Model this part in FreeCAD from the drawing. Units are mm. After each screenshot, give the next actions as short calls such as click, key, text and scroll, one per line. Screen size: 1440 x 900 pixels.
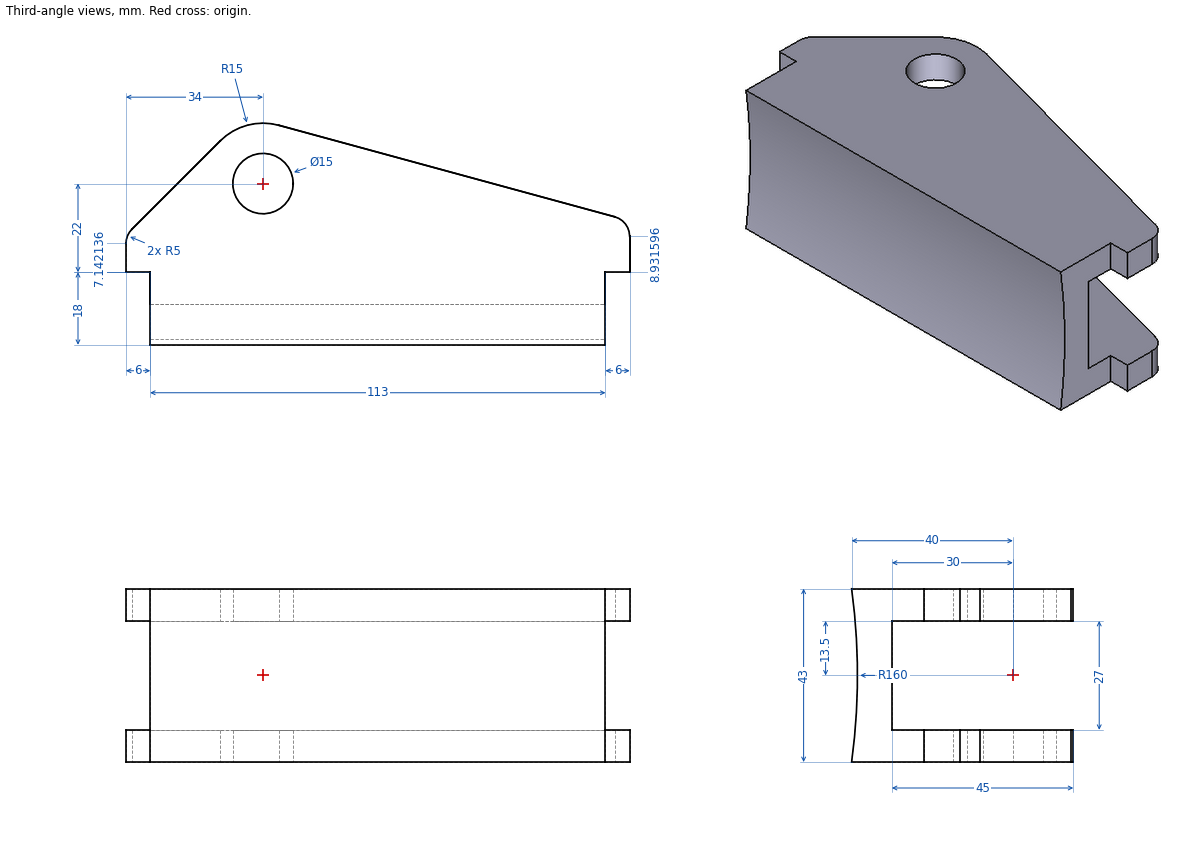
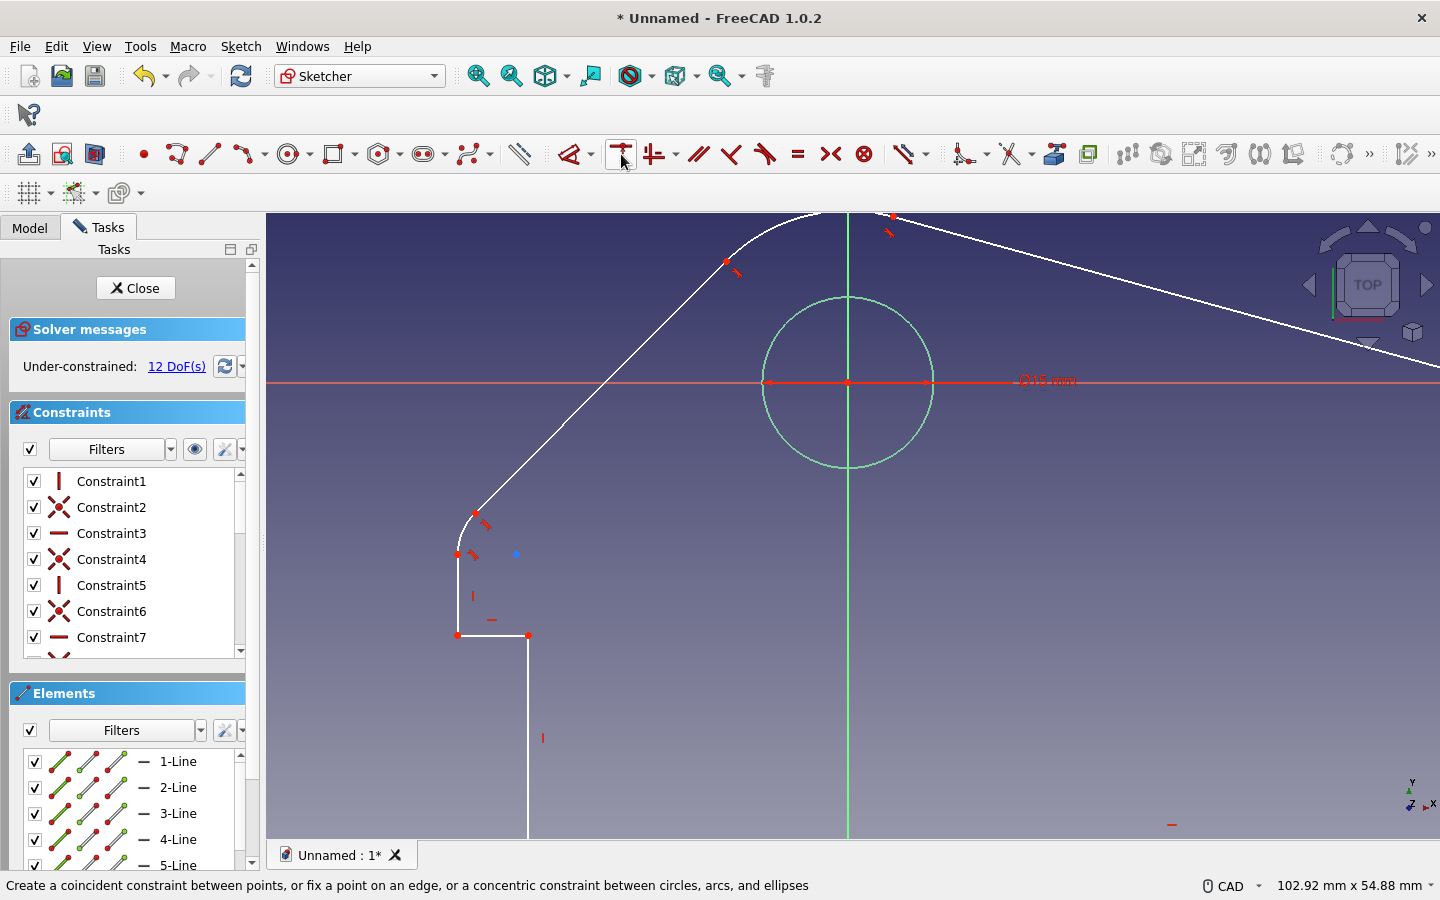
scroll(468, 524, down, 4)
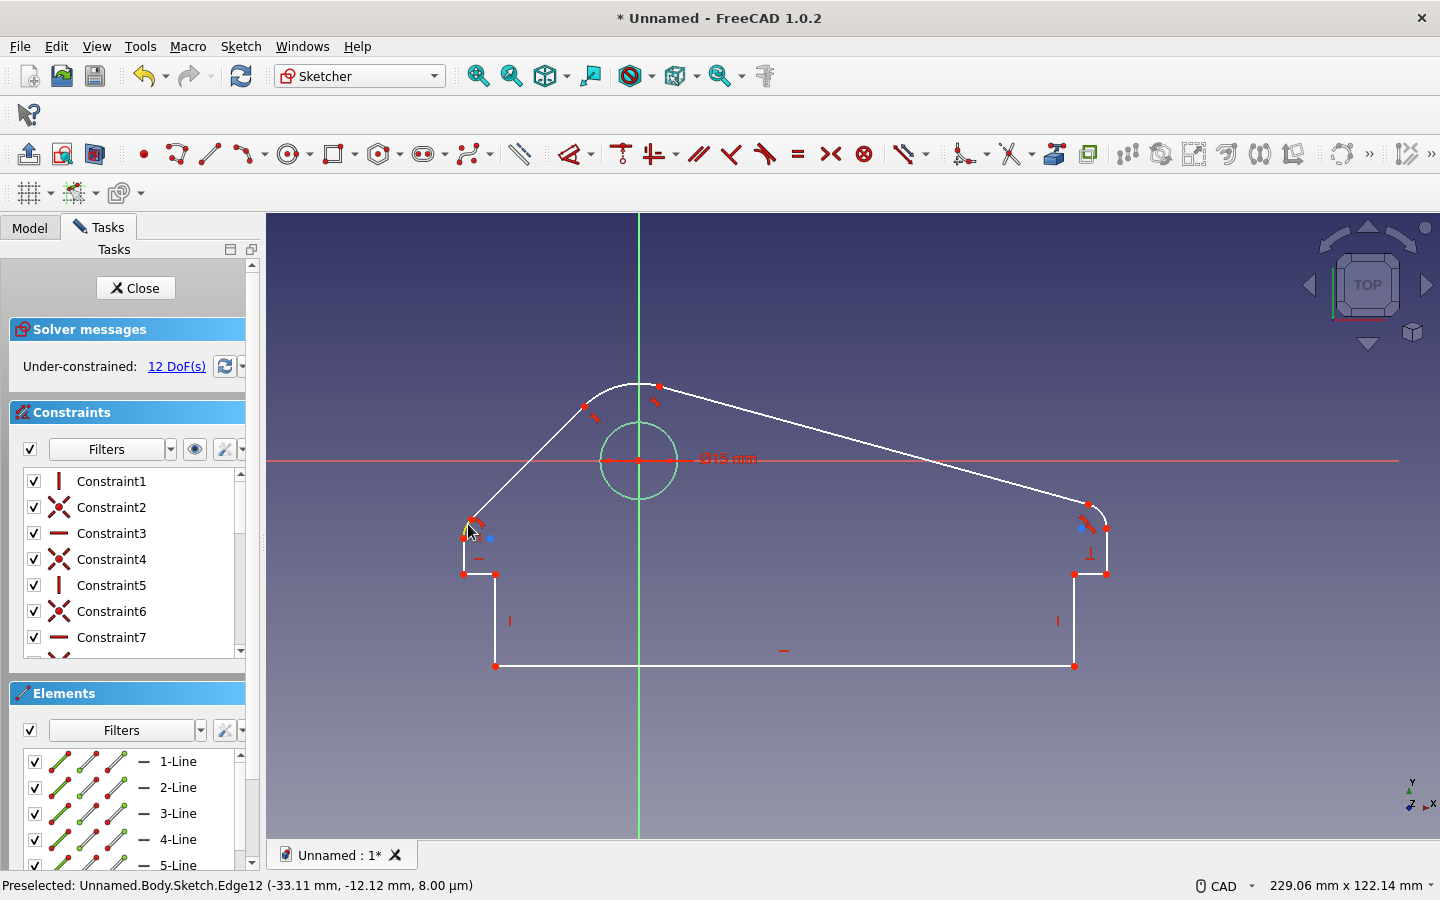
scroll(1105, 519, up, 2)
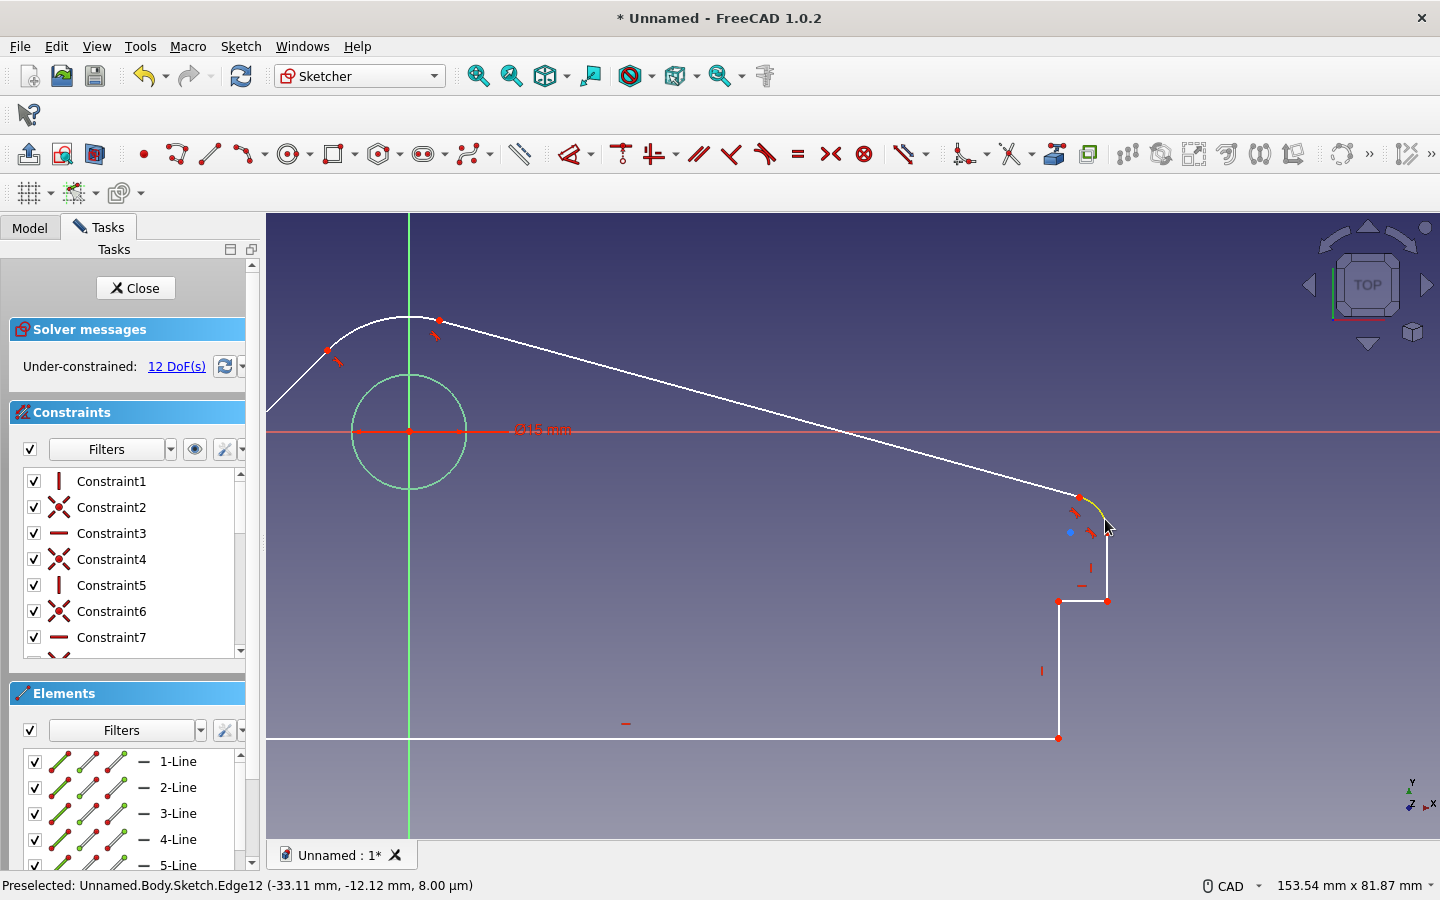
click(1104, 519)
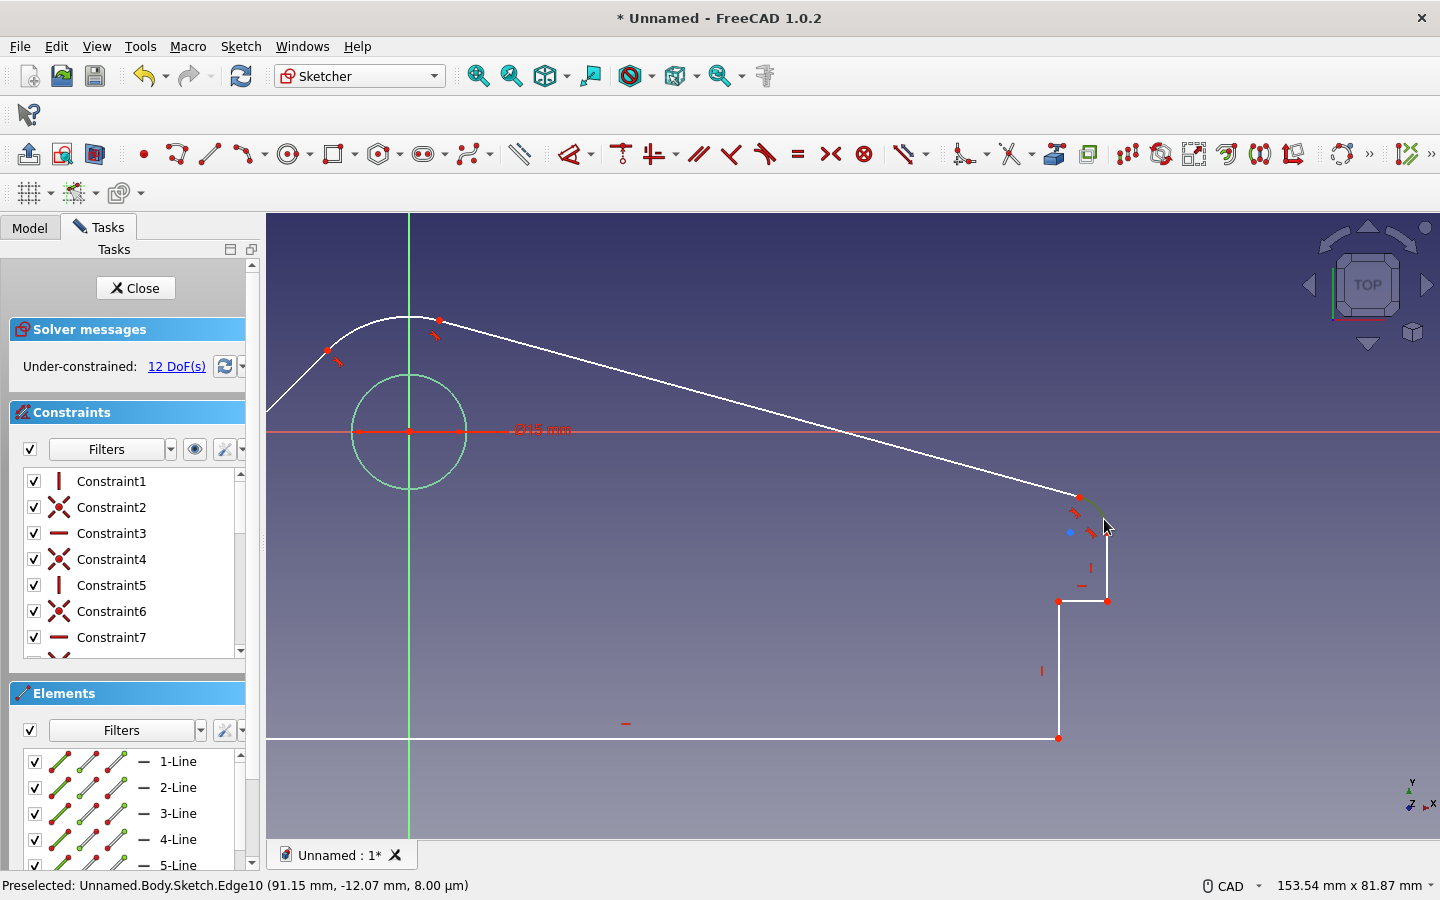
scroll(1105, 519, down, 2)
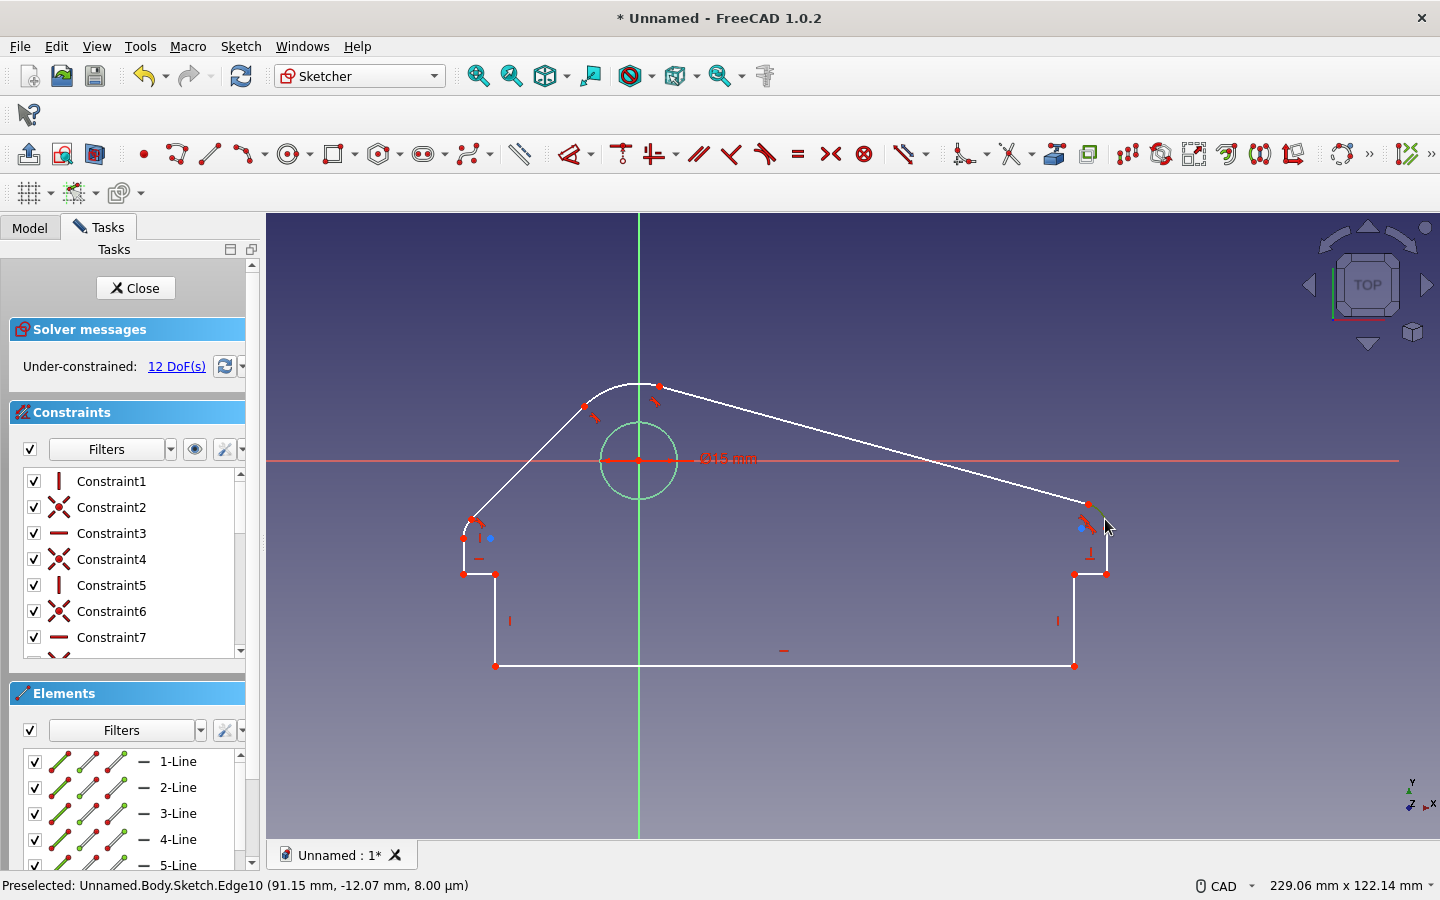
scroll(467, 524, up, 4)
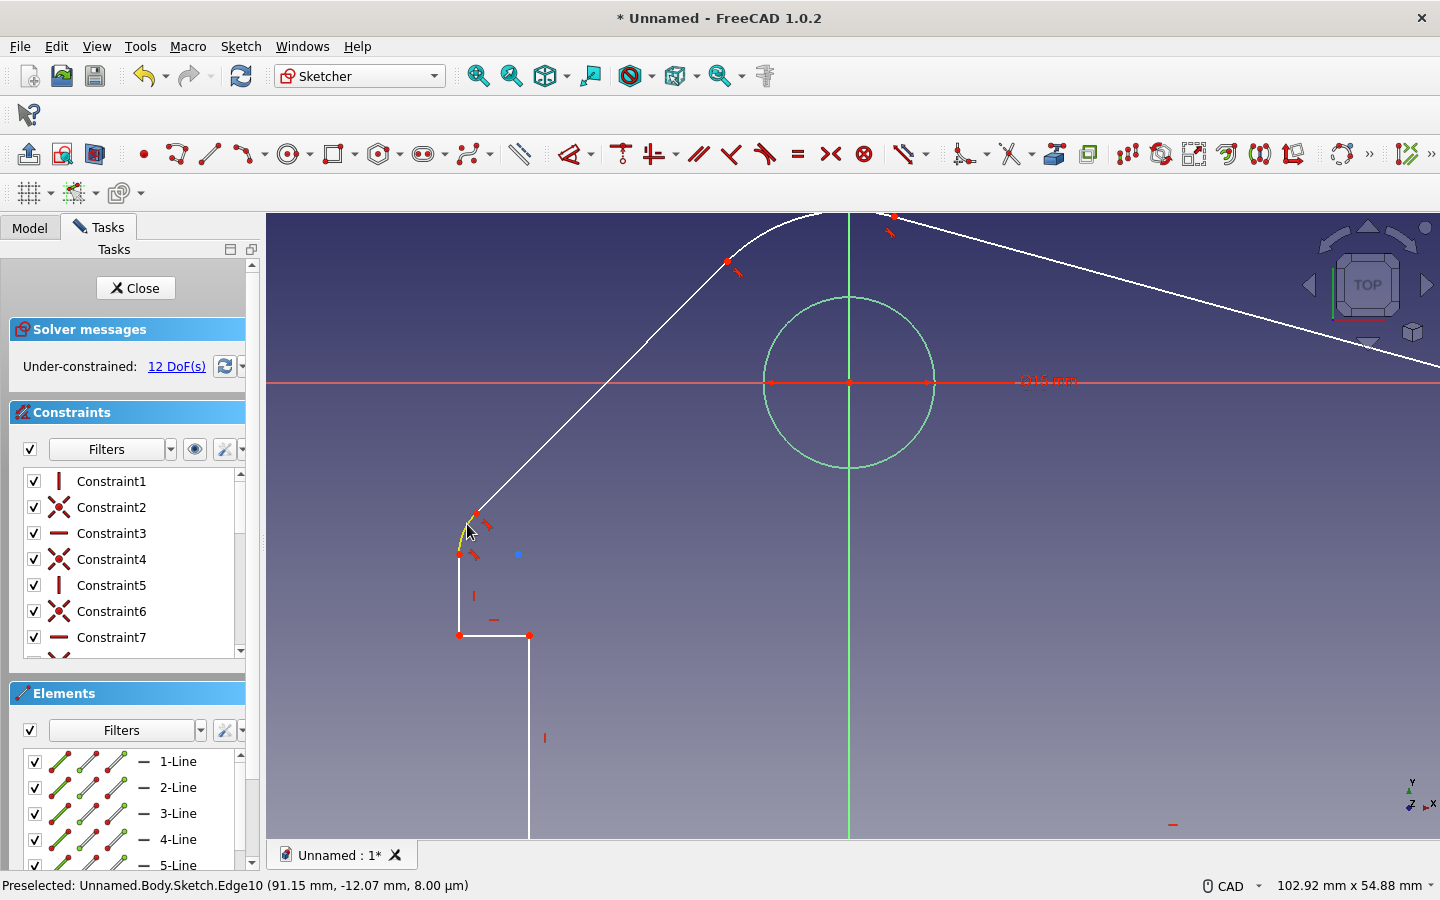
click(468, 524)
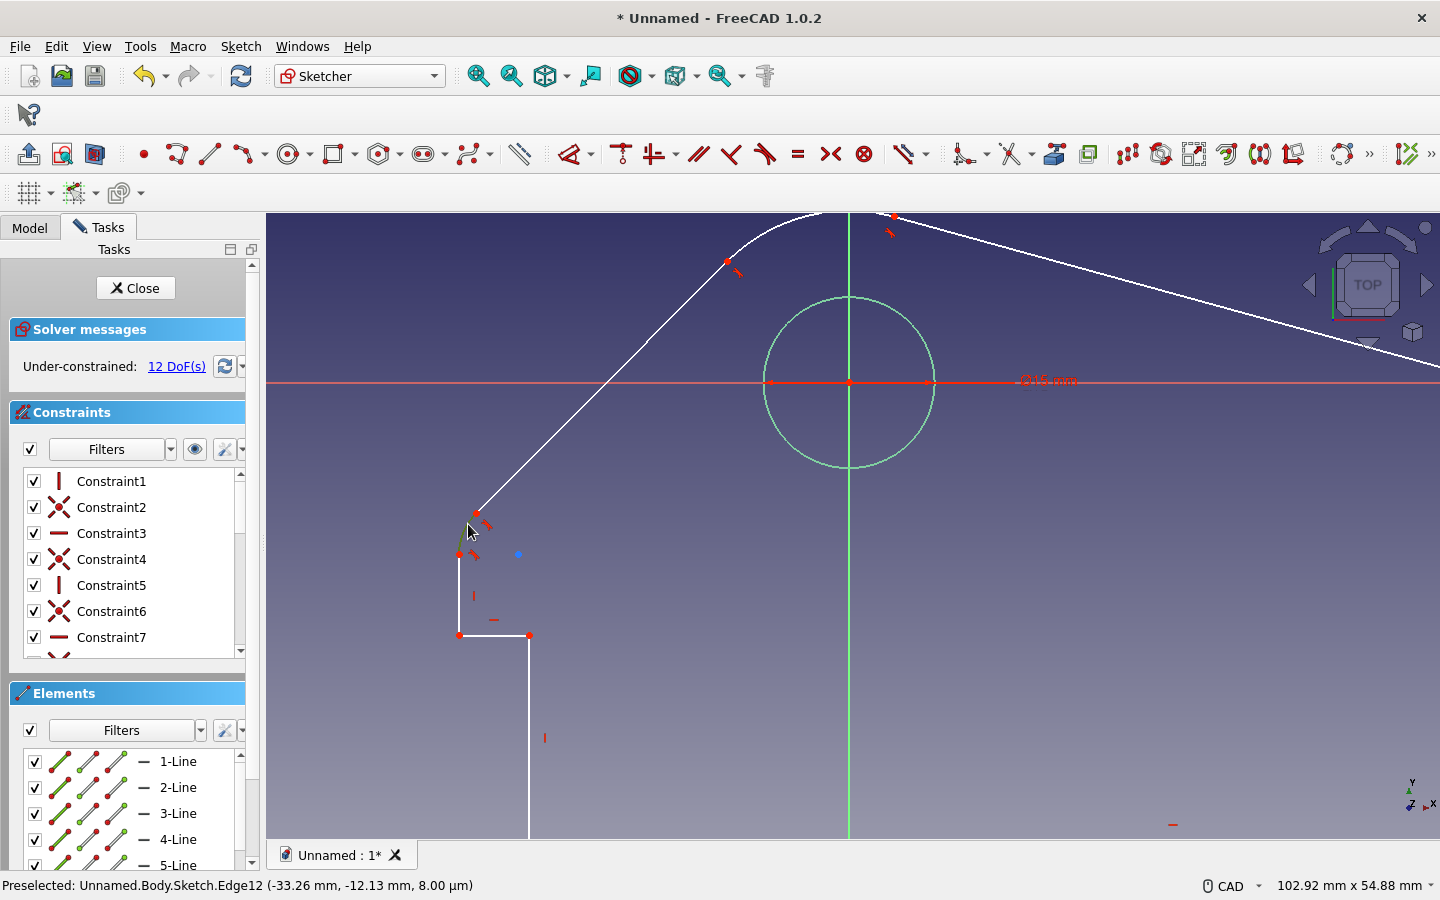
key(e)